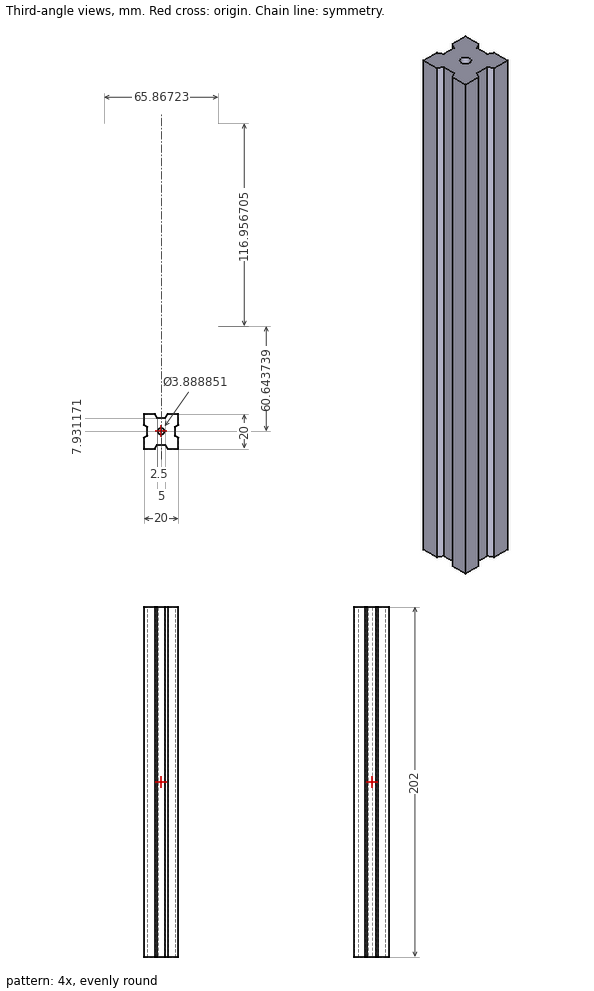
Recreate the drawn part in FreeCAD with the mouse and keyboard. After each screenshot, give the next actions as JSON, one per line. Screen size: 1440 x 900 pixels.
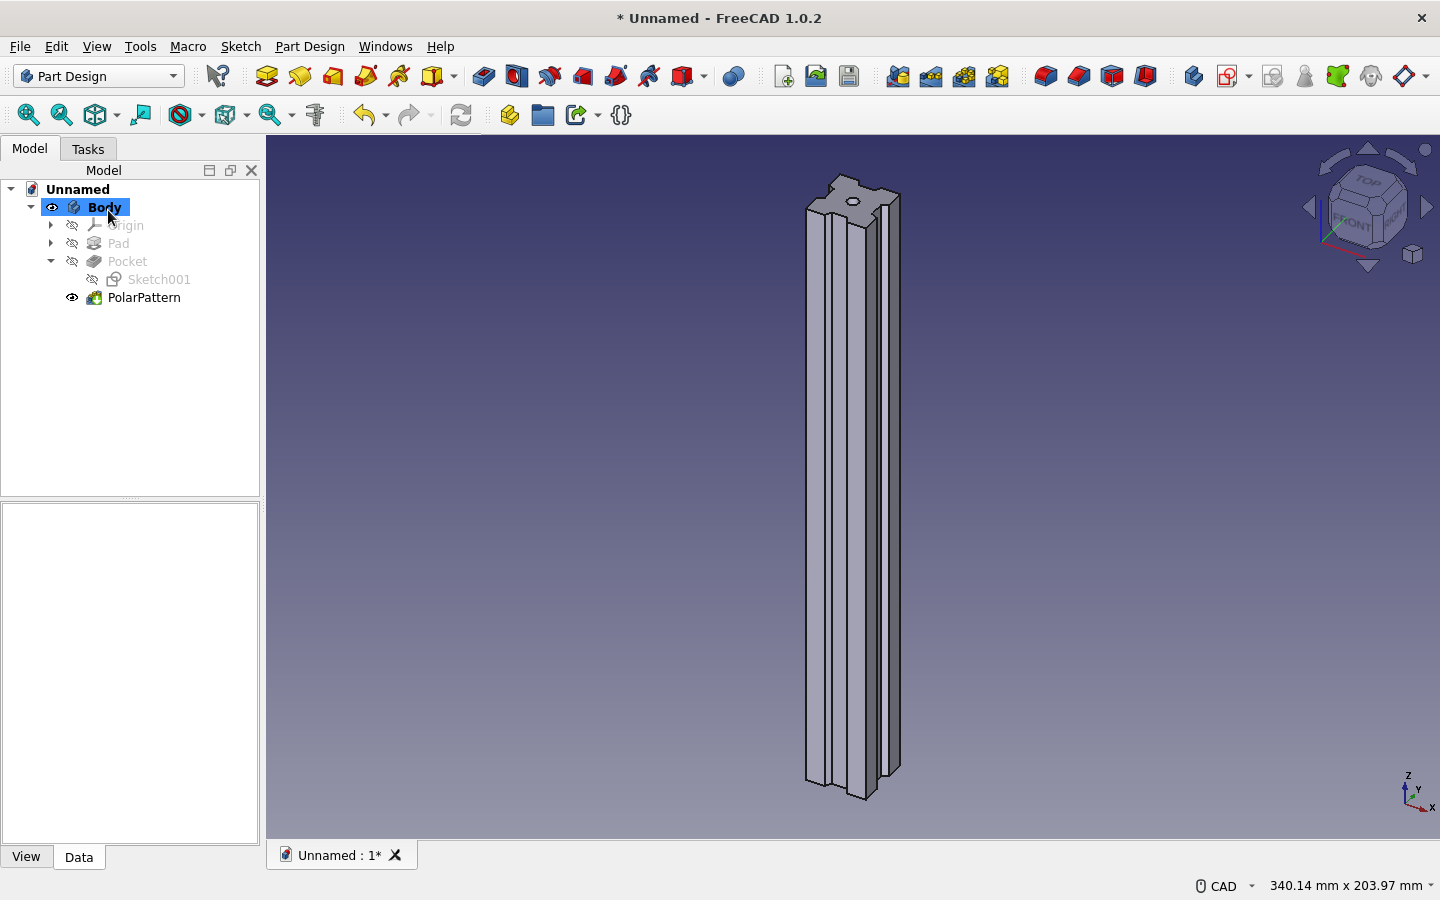
{"action": "key", "text": "0"}